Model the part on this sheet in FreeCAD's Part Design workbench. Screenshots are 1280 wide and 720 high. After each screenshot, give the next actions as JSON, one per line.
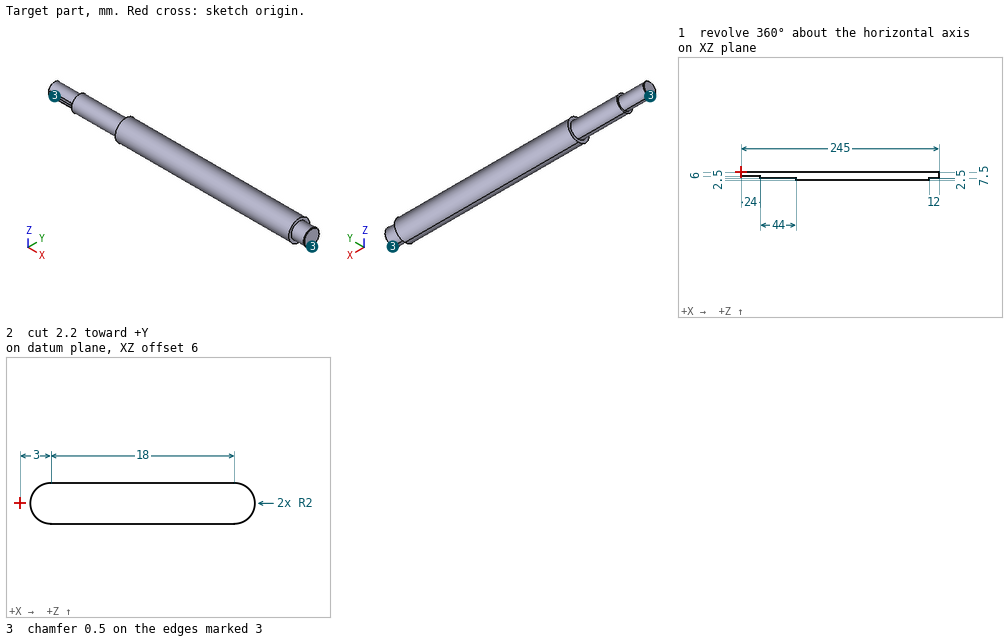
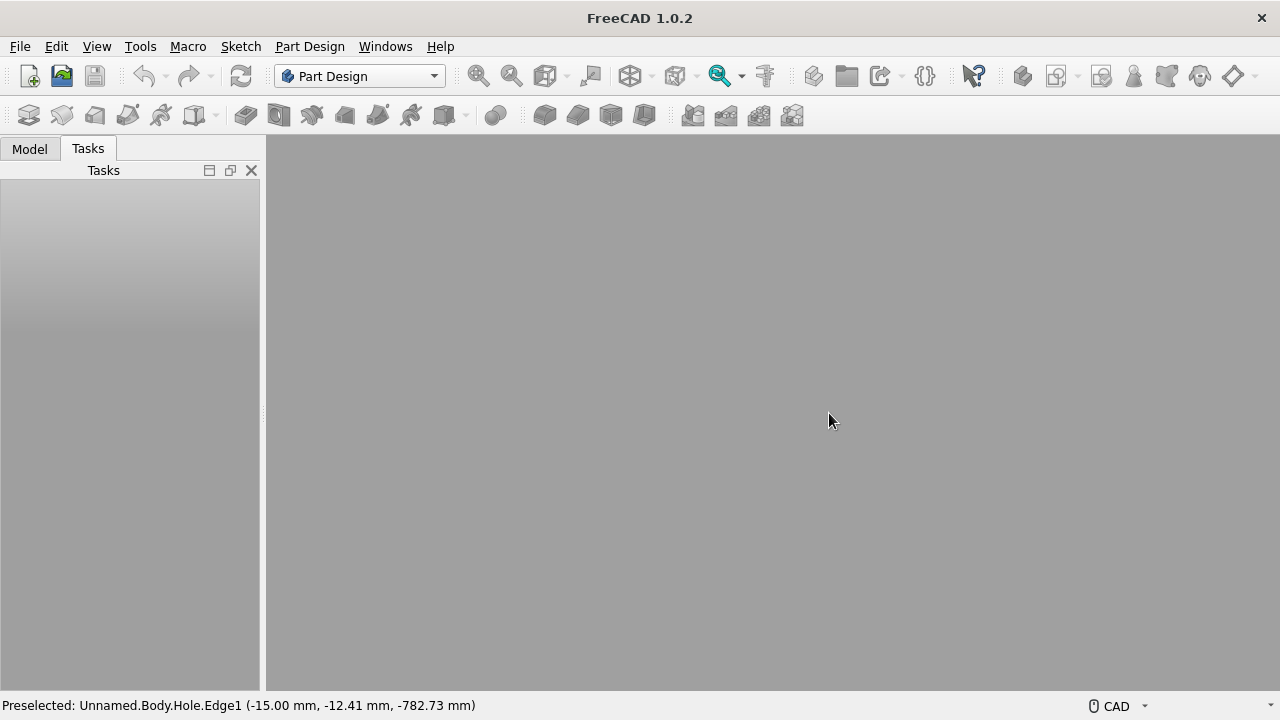
{"action": "left_click", "coordinate": [29, 76]}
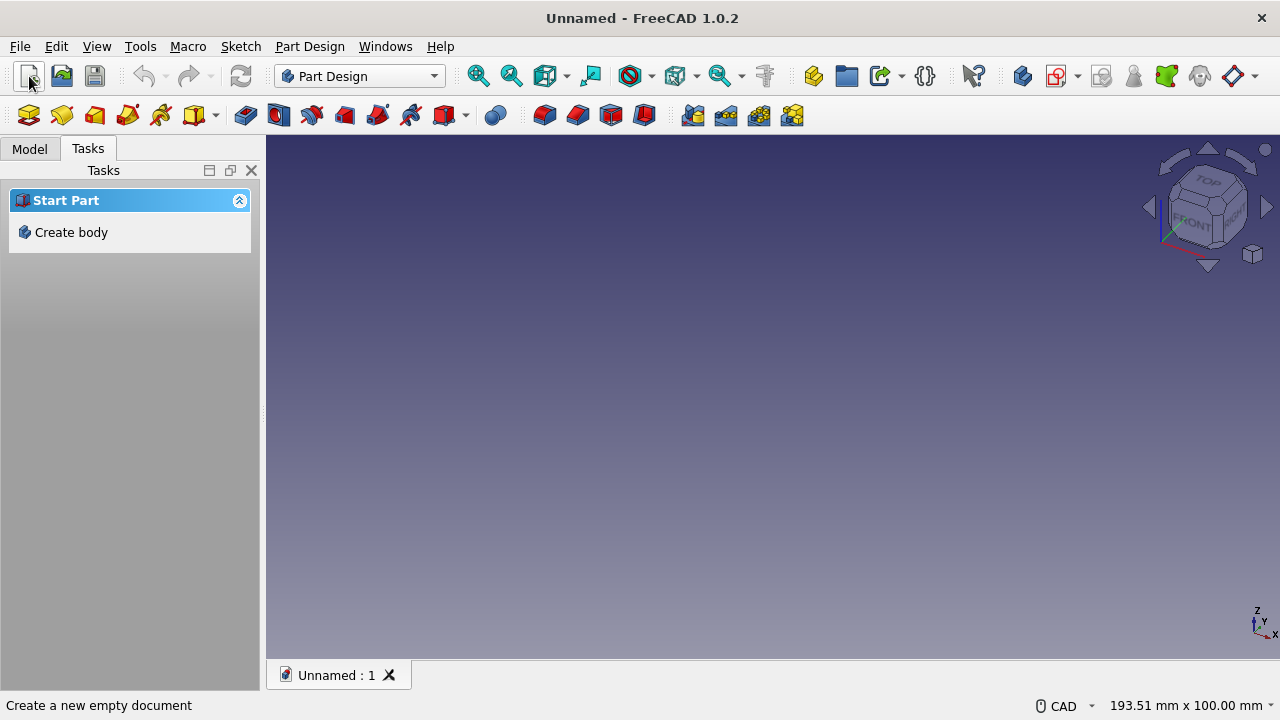
{"action": "left_click", "coordinate": [1056, 76]}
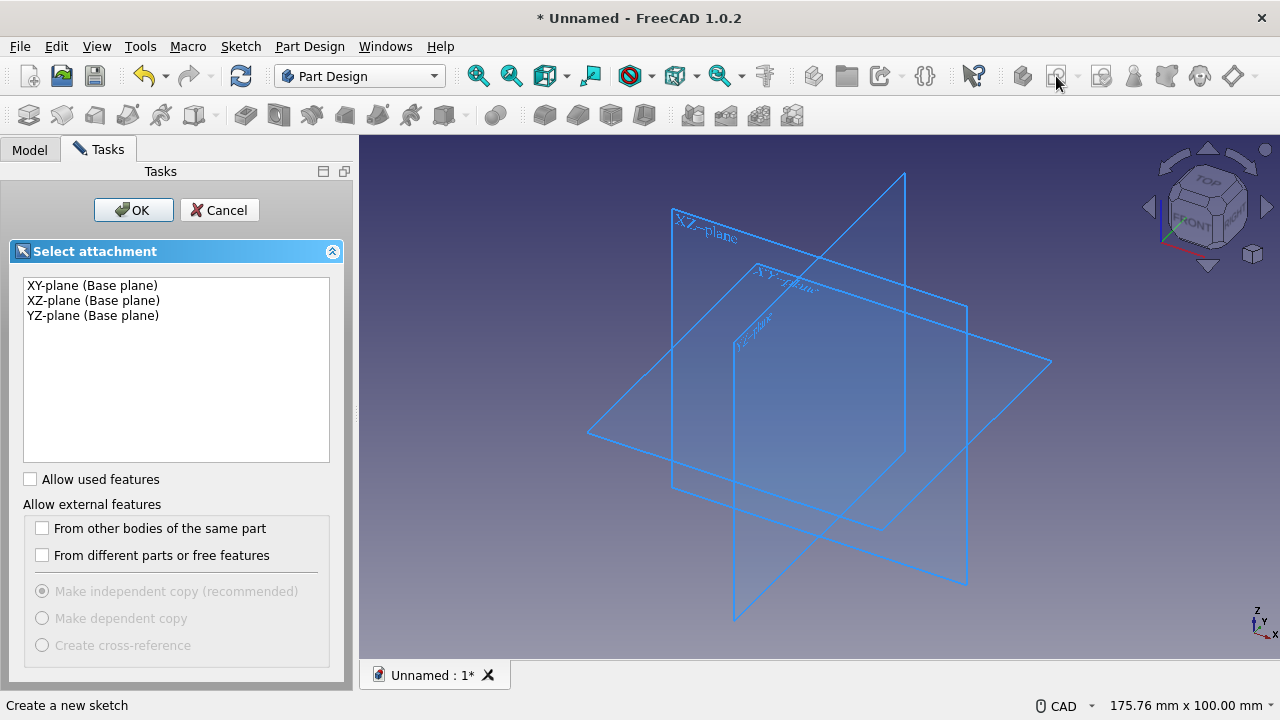
{"action": "left_click", "coordinate": [84, 300]}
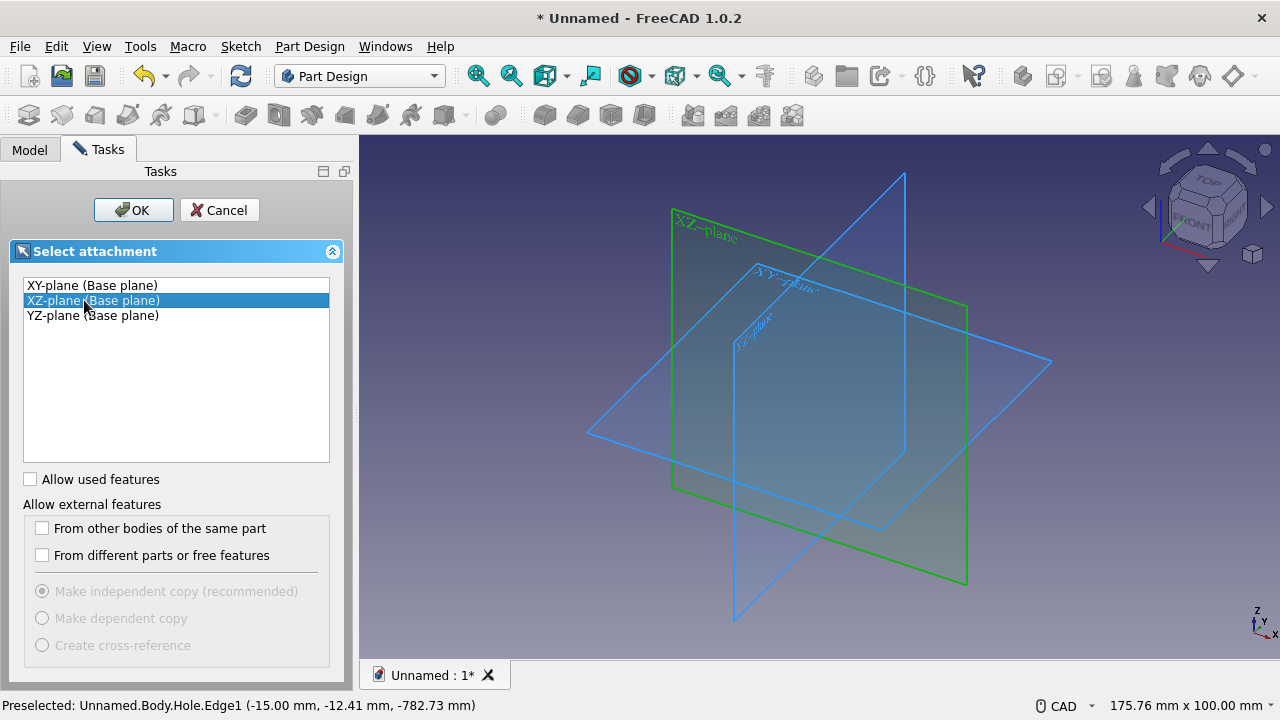
{"action": "left_click", "coordinate": [134, 210]}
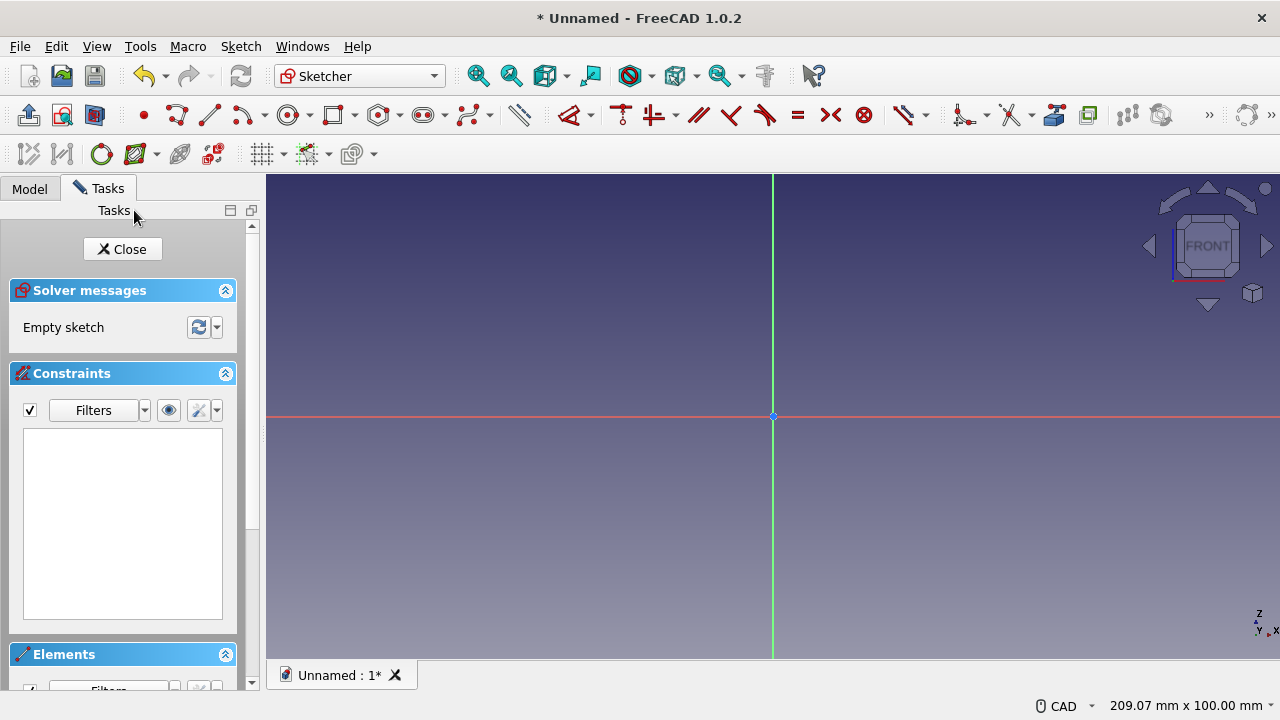
{"action": "scroll", "coordinate": [294, 397], "scroll_direction": "down", "scroll_amount": 4}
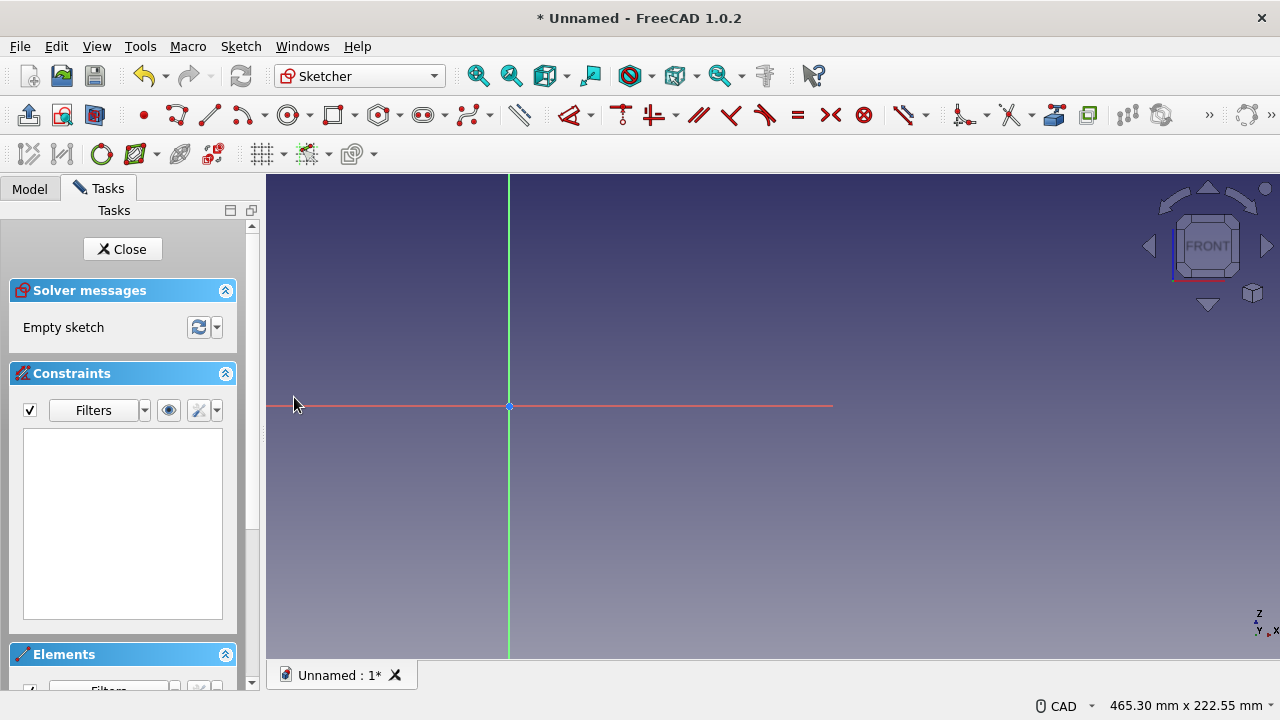
{"action": "left_click", "coordinate": [177, 116]}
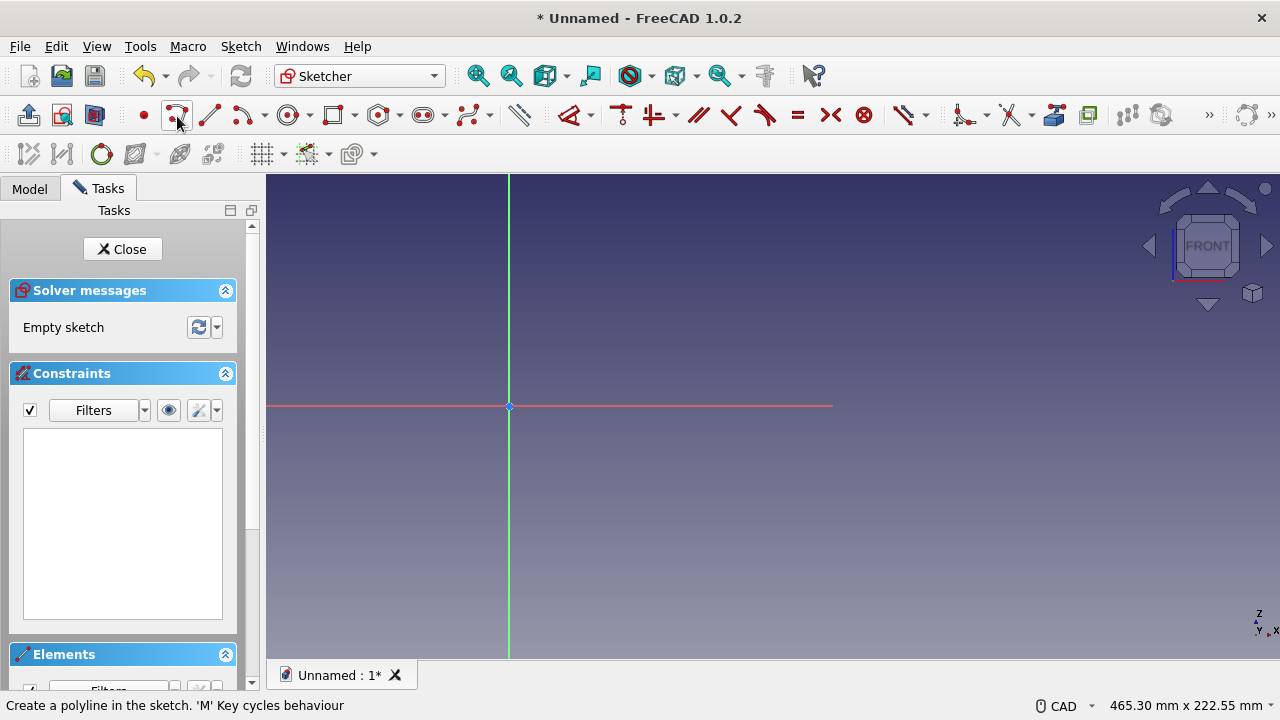
{"action": "left_click", "coordinate": [509, 406]}
{"action": "left_click", "coordinate": [1043, 415]}
{"action": "left_click", "coordinate": [1043, 422]}
{"action": "left_click", "coordinate": [1017, 422]}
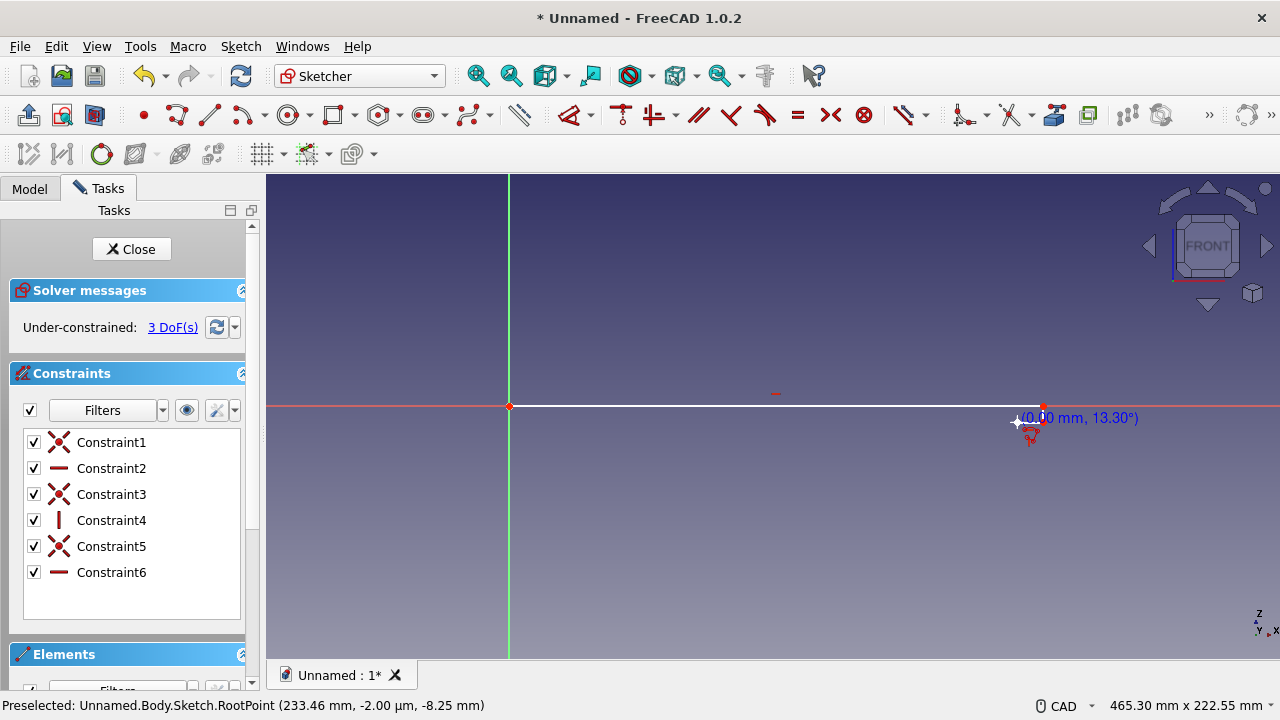
{"action": "scroll", "coordinate": [1017, 428], "scroll_direction": "up", "scroll_amount": 6}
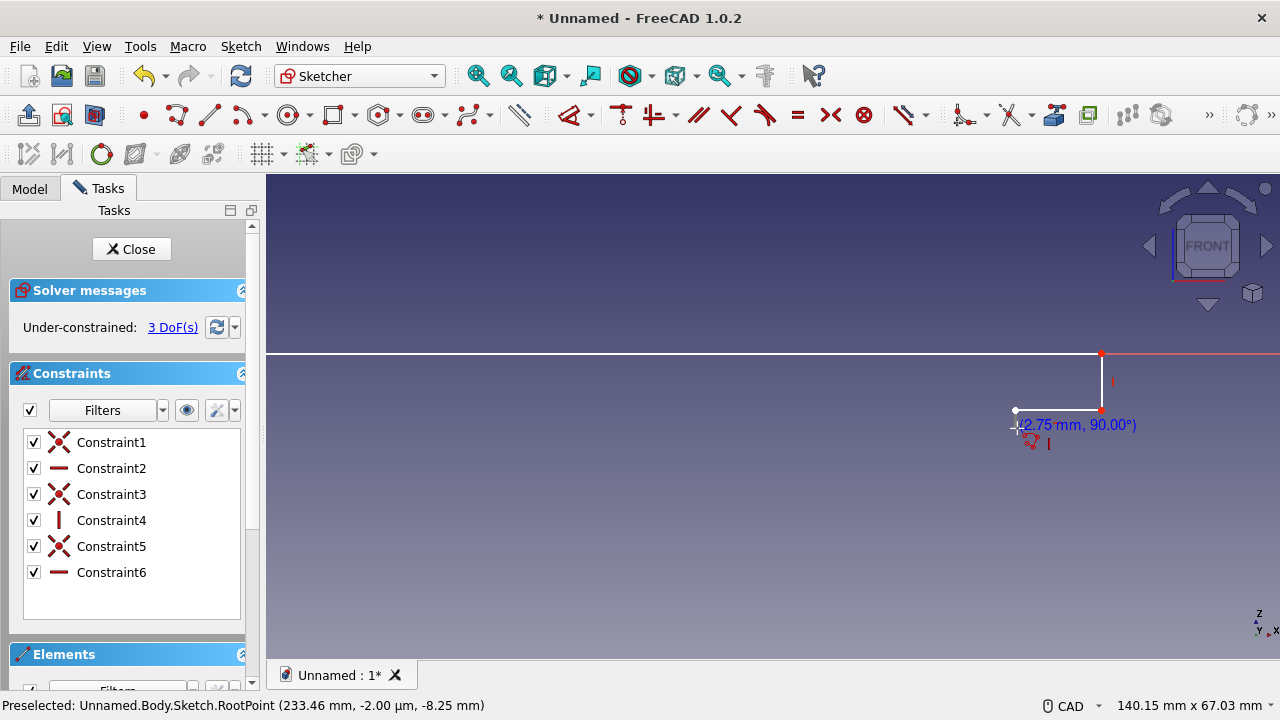
{"action": "left_click", "coordinate": [1015, 426]}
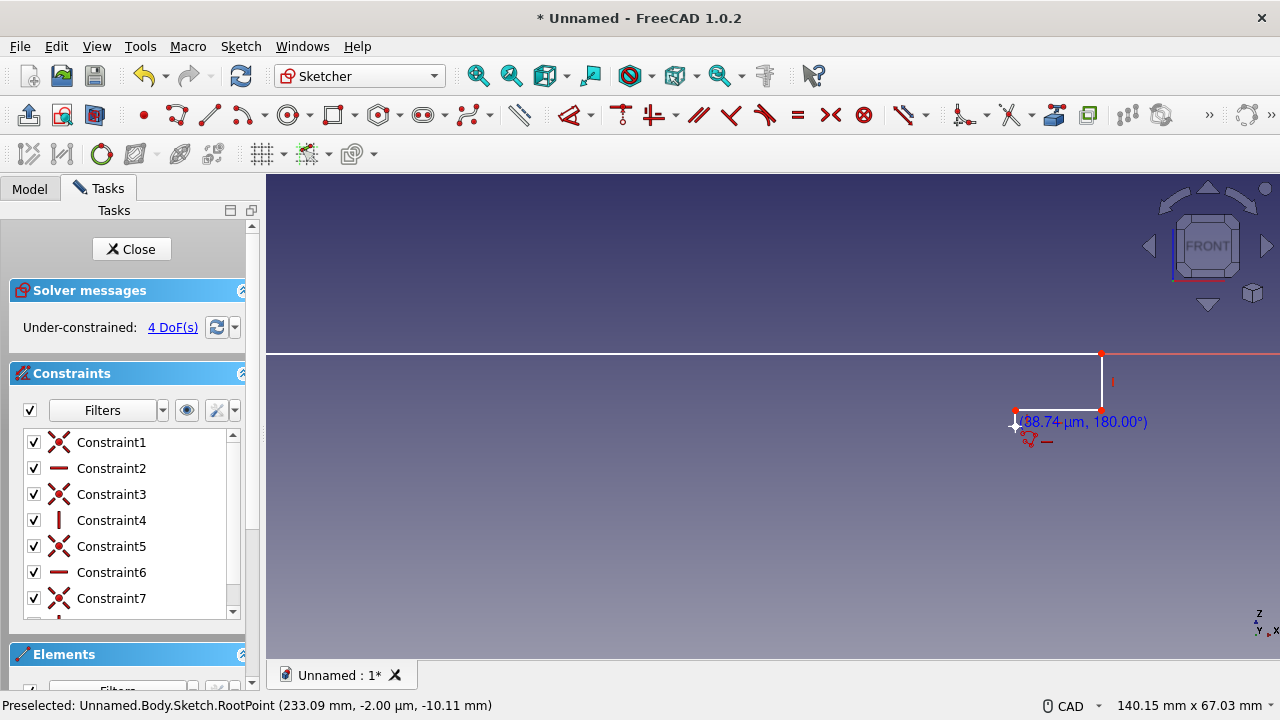
{"action": "scroll", "coordinate": [915, 428], "scroll_direction": "down", "scroll_amount": 6}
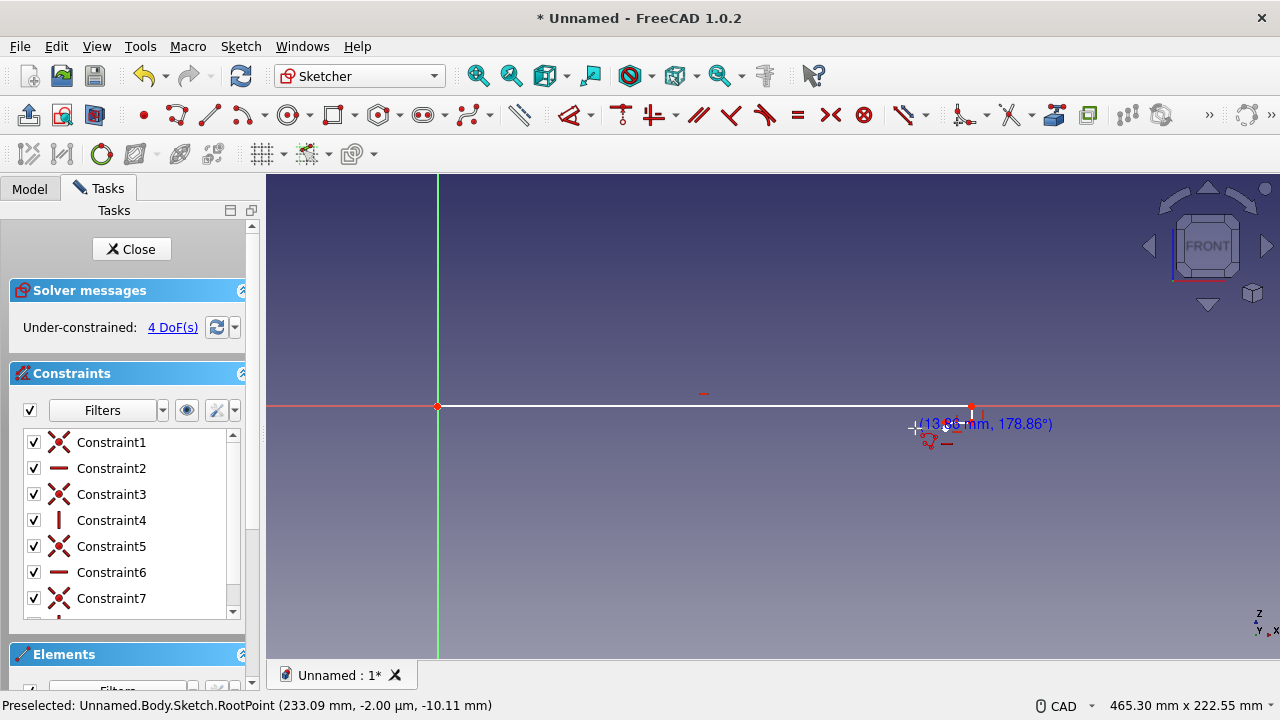
{"action": "left_click", "coordinate": [586, 428]}